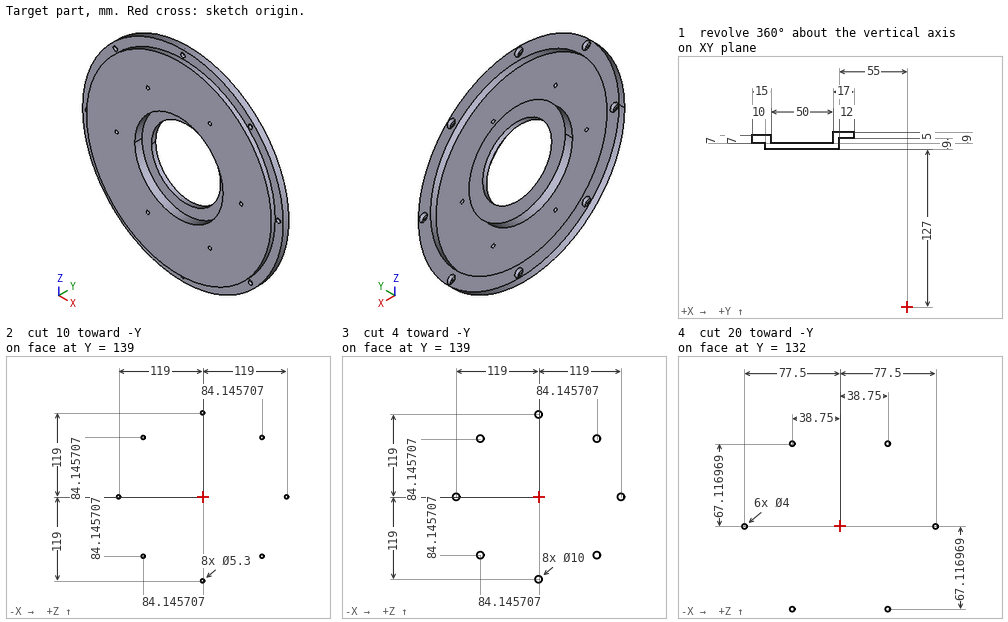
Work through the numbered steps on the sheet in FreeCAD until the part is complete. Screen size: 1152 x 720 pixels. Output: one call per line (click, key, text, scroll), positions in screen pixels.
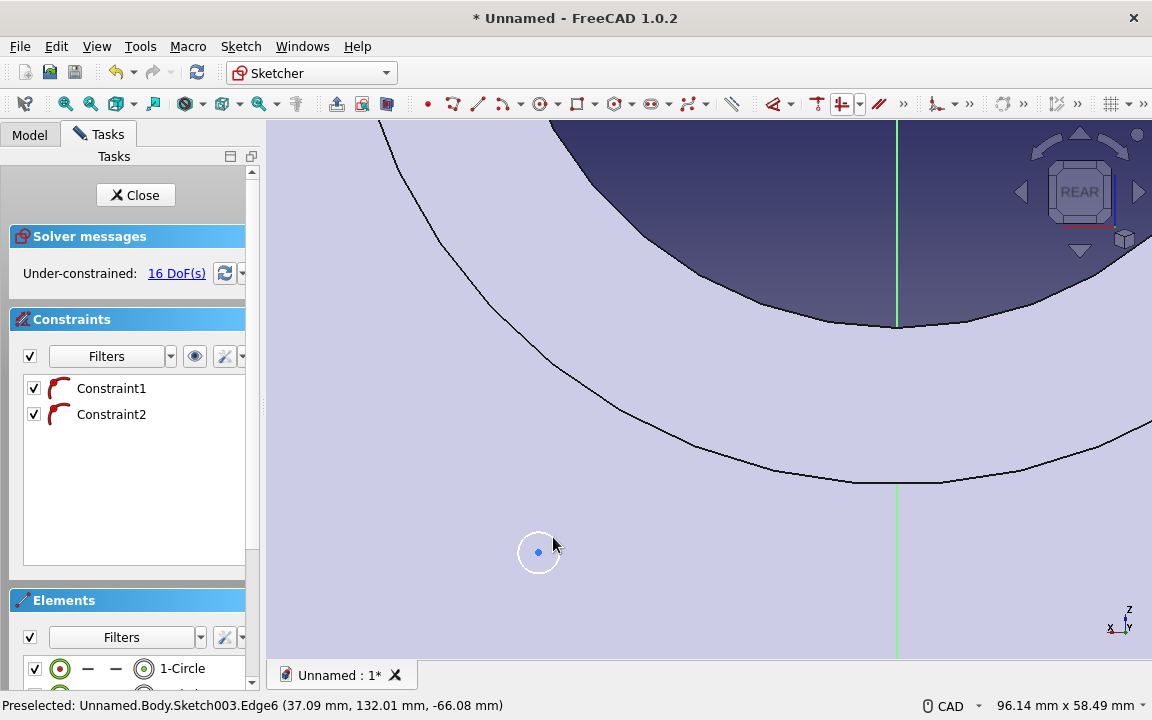
scroll(556, 539, down, 7)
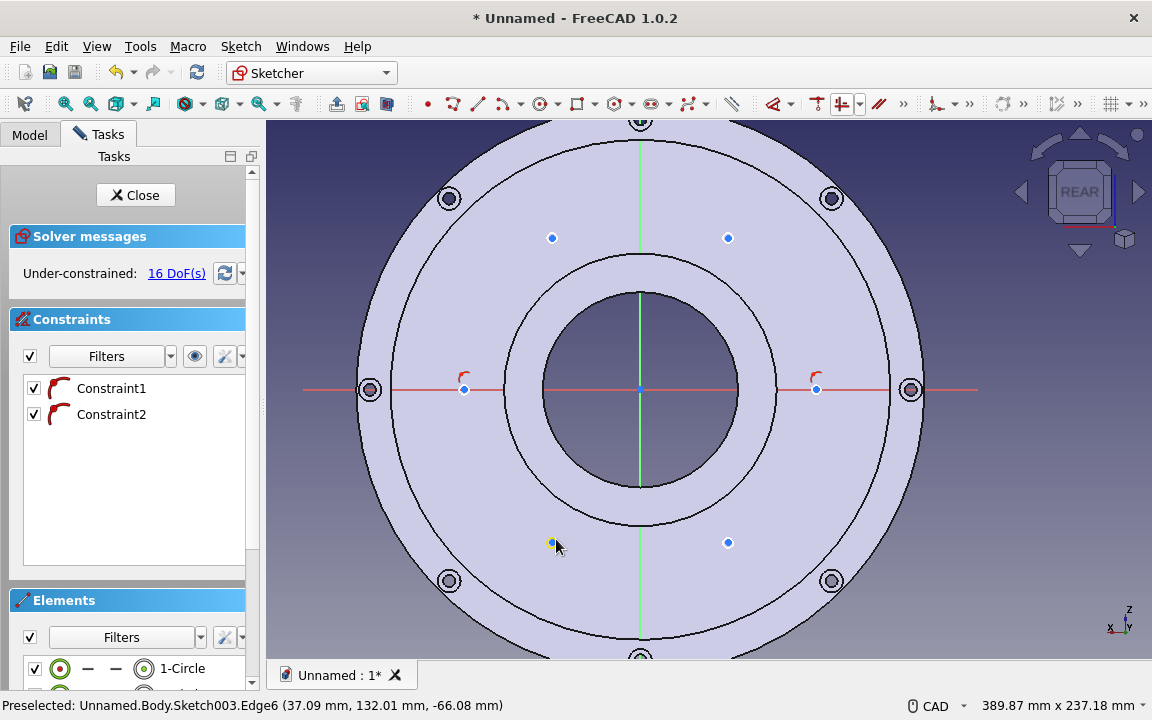
scroll(467, 386, up, 8)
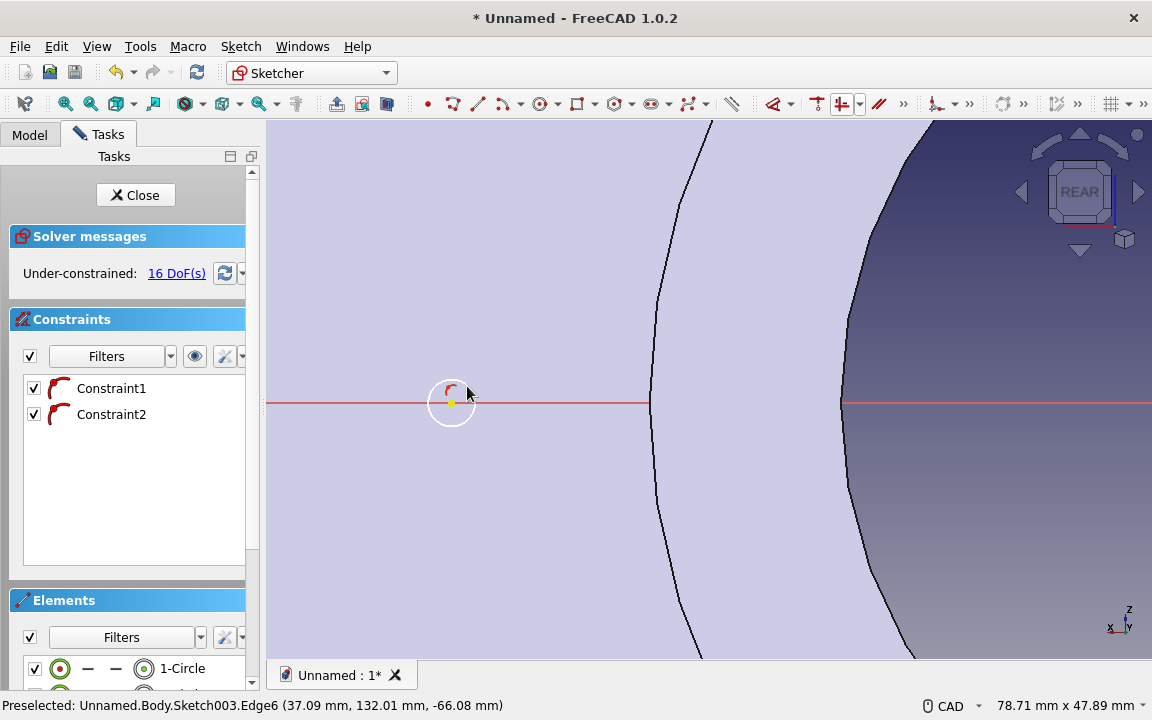
click(468, 386)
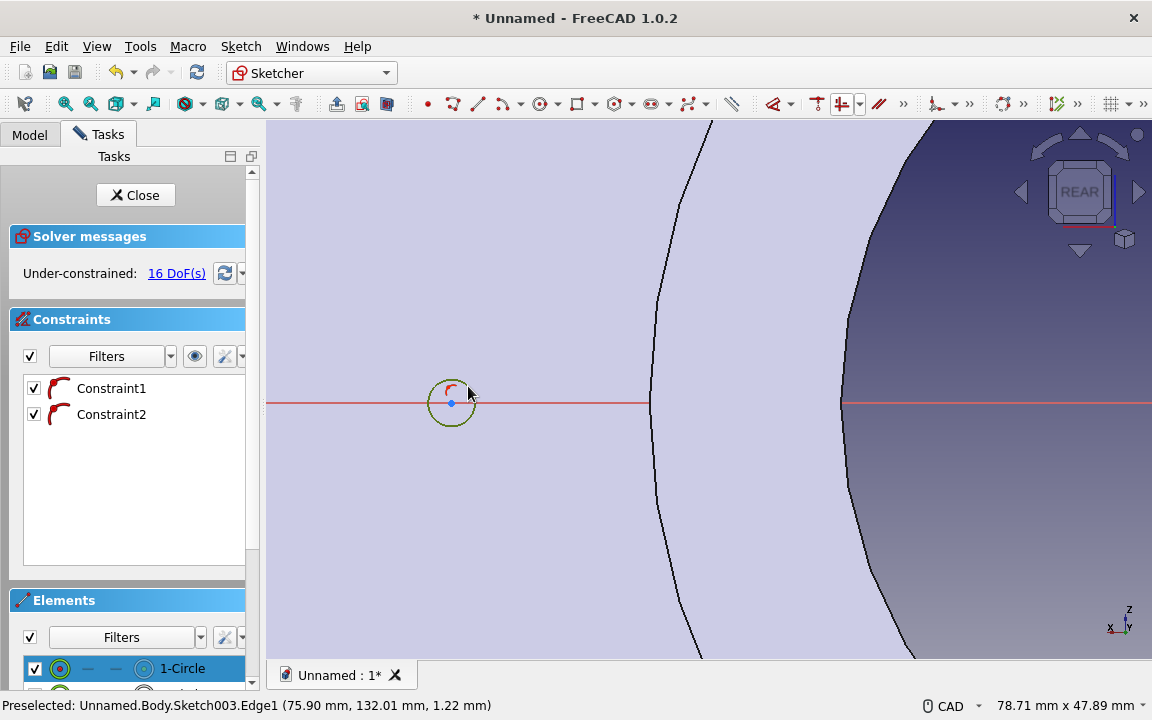
scroll(467, 386, down, 8)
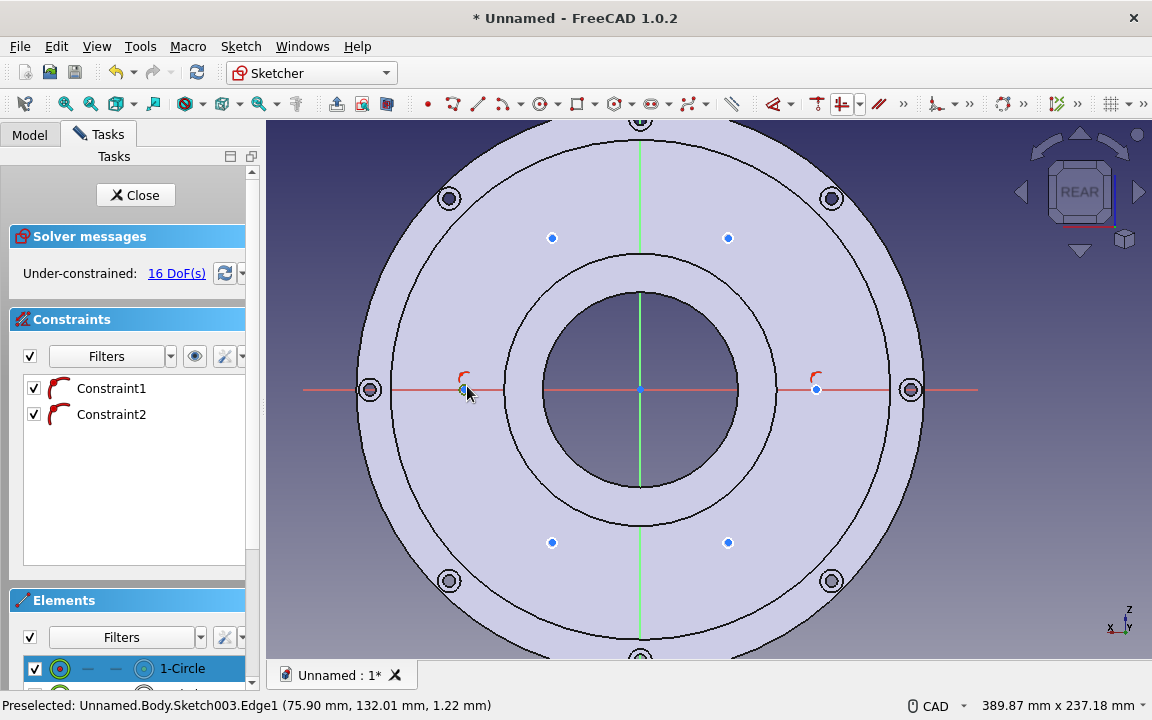
scroll(556, 235, up, 6)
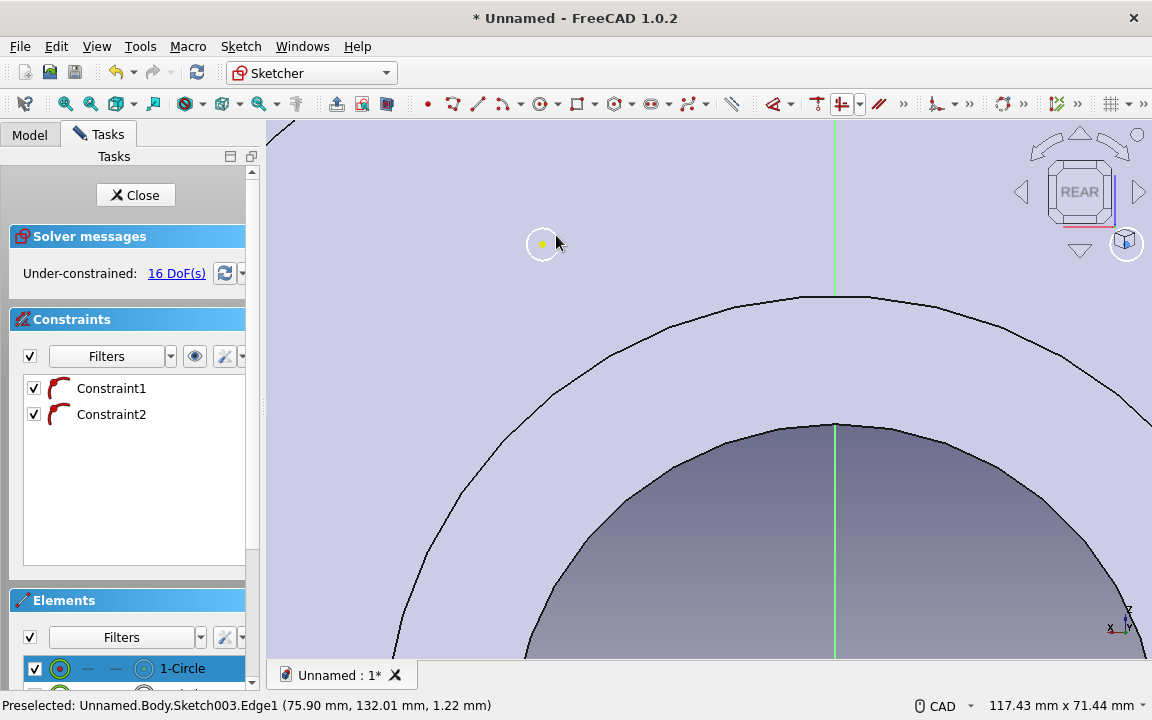
click(554, 233)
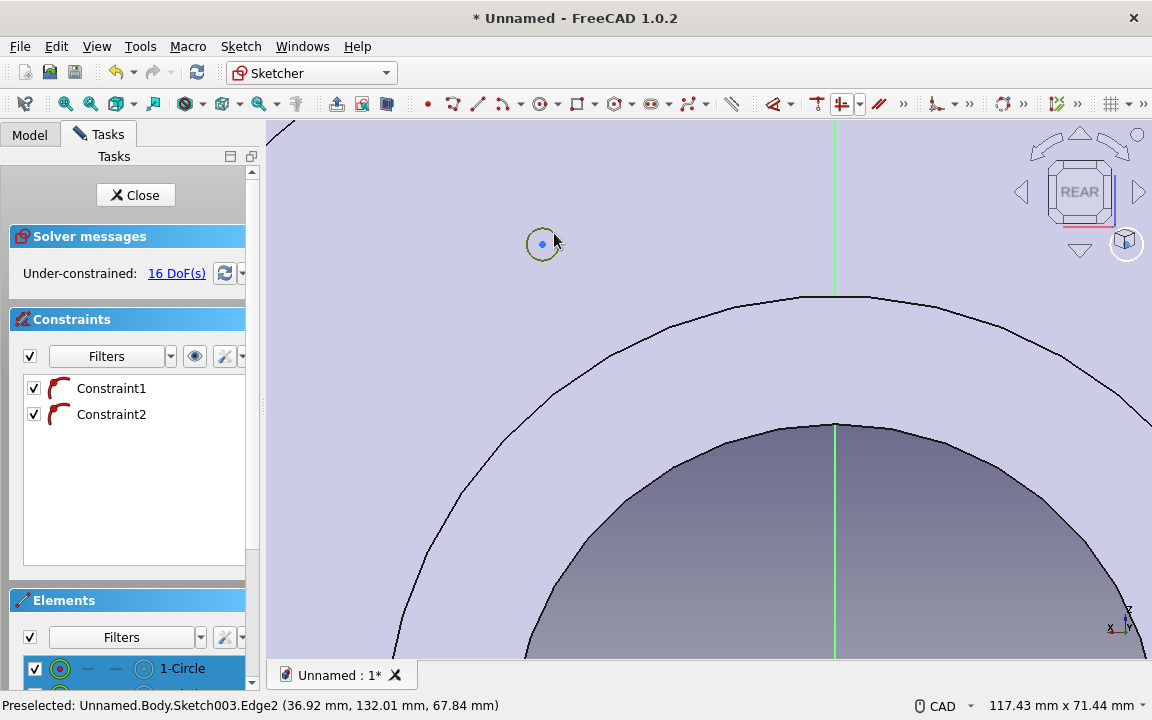
scroll(556, 235, down, 6)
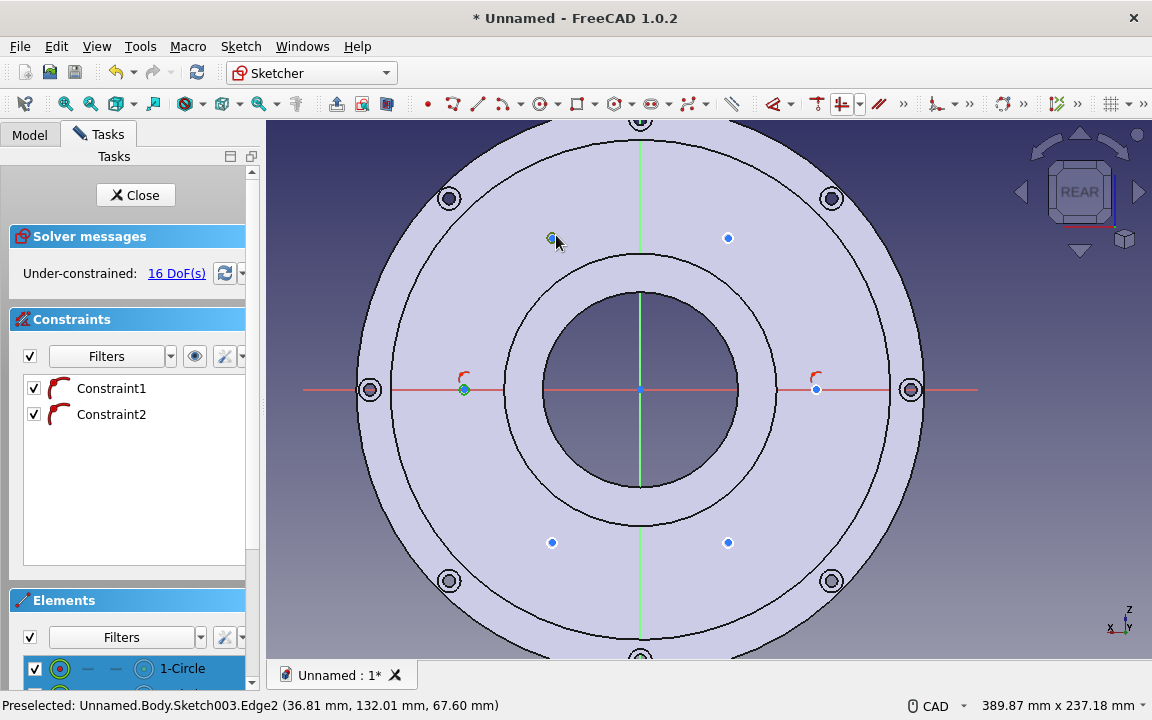
scroll(732, 234, up, 6)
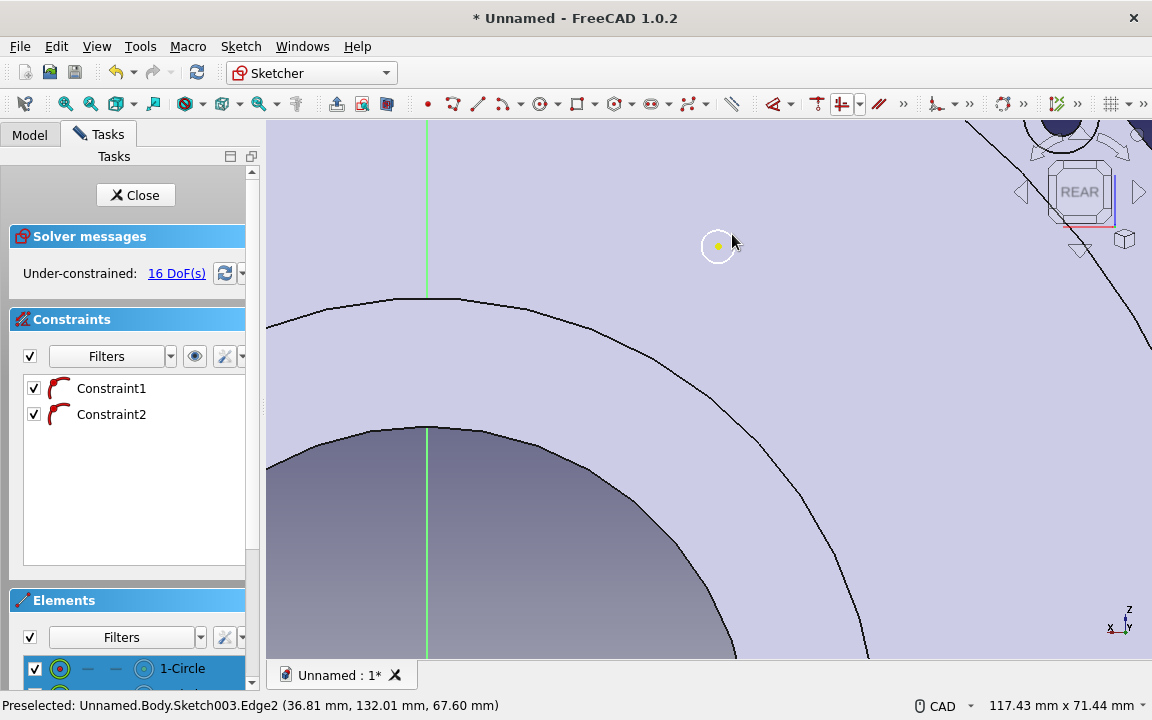
click(730, 235)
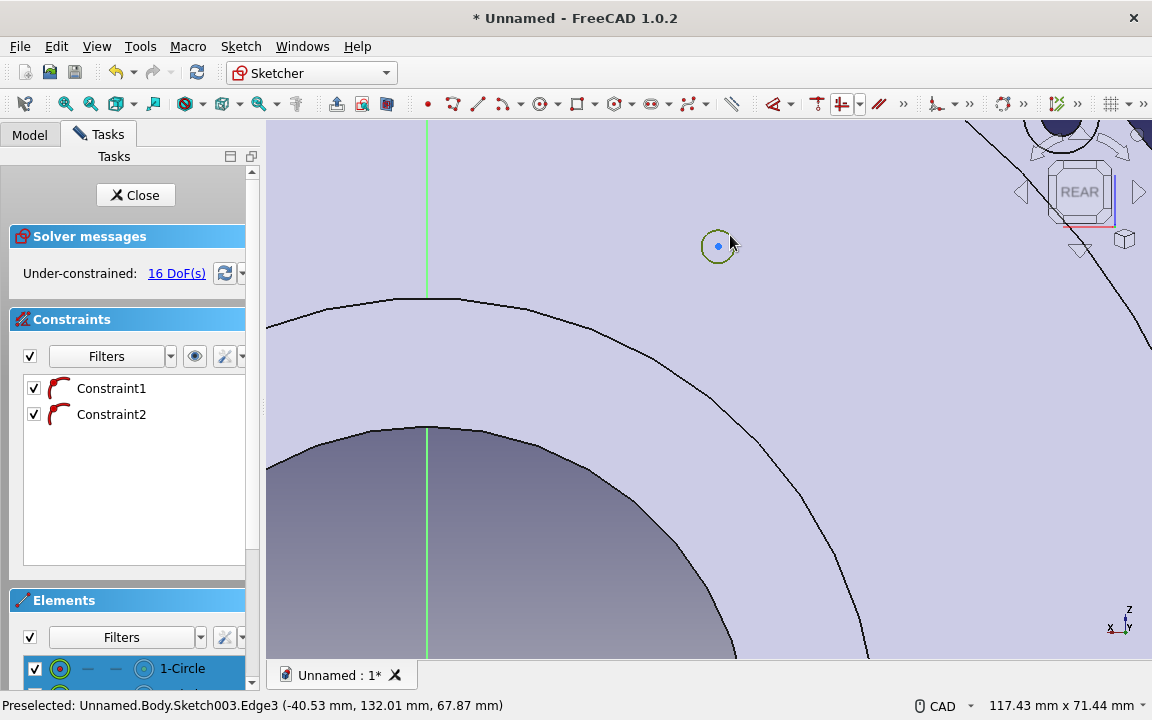
scroll(733, 234, down, 6)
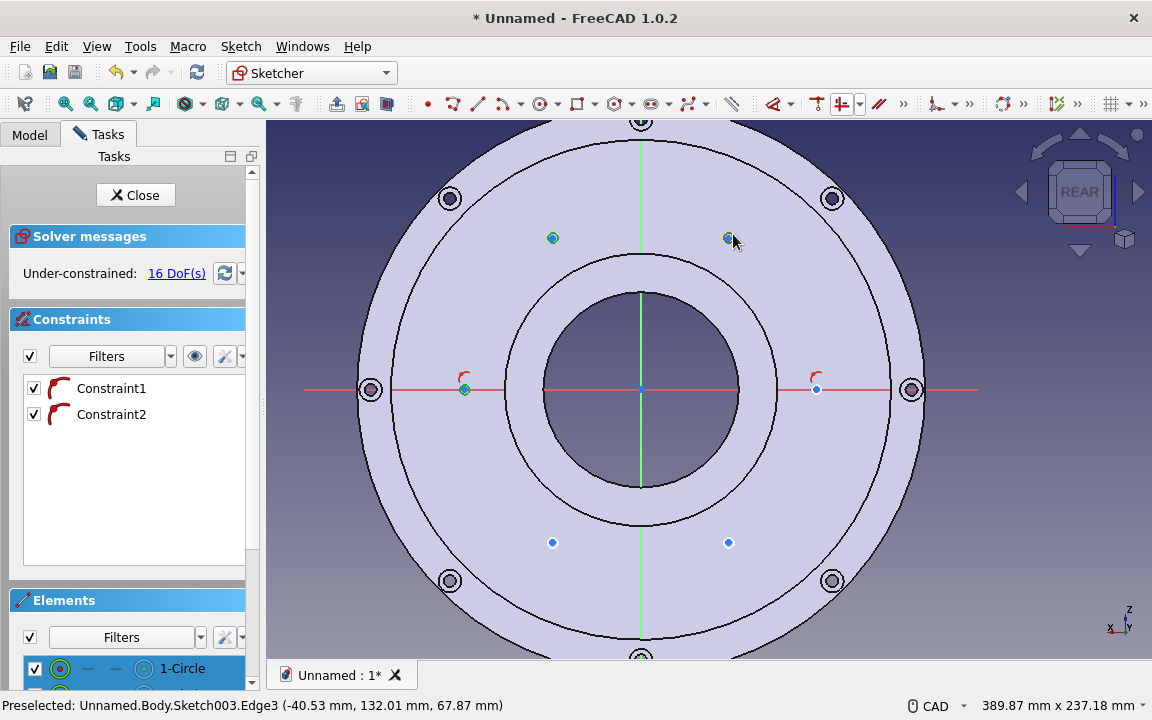
scroll(820, 387, up, 8)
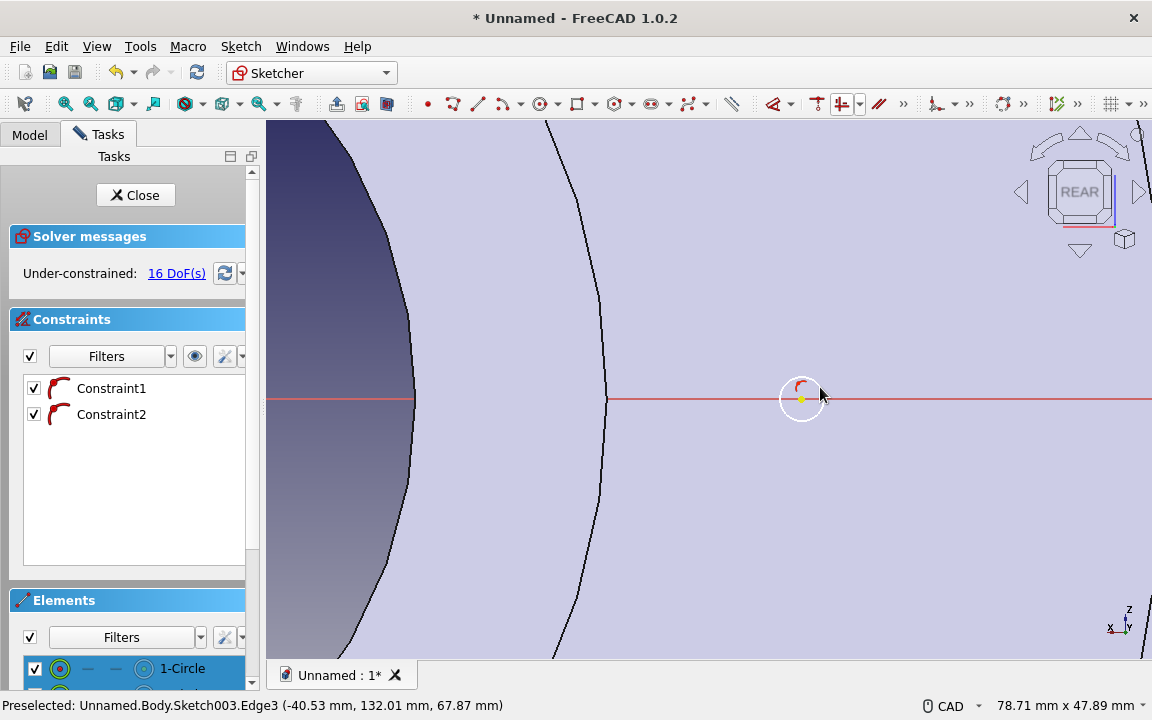
click(817, 384)